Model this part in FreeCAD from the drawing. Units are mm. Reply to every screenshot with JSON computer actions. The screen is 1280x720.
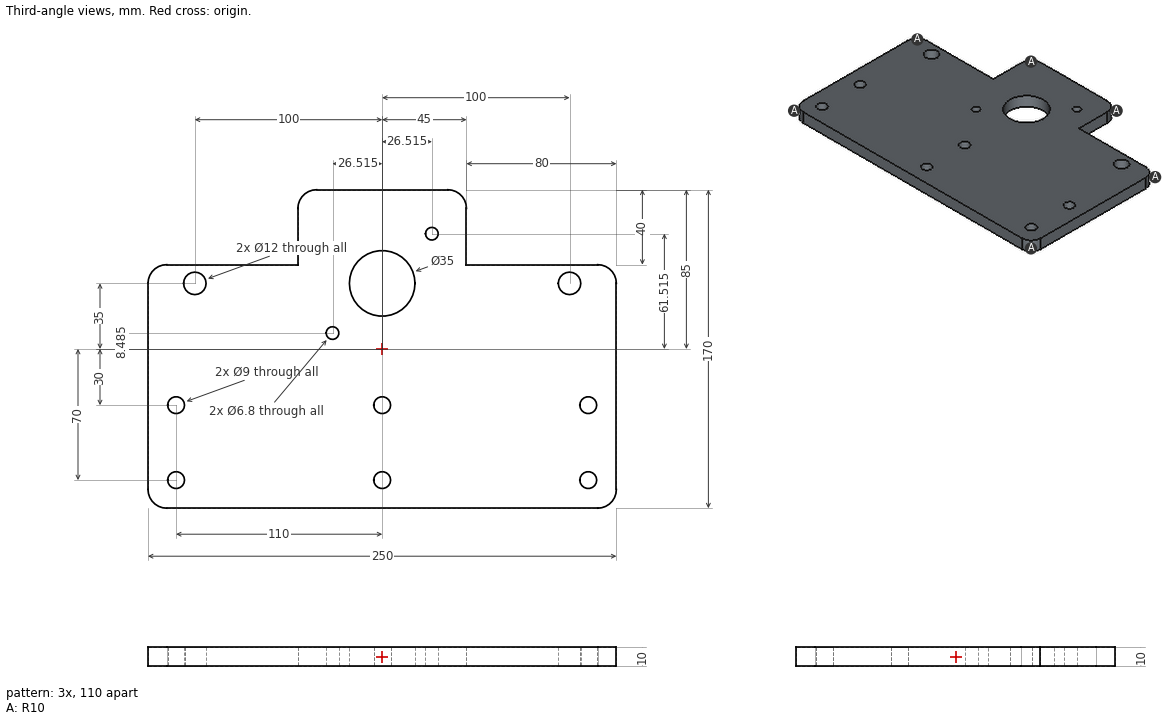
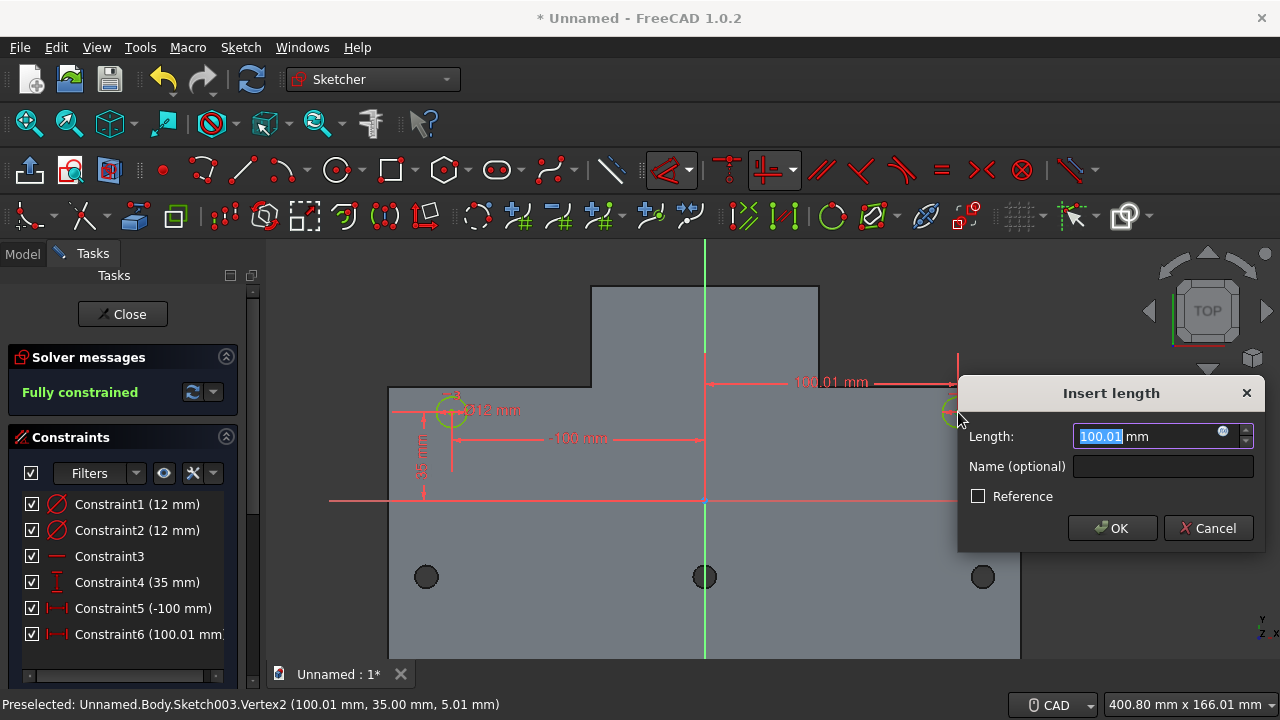
{"action": "type", "text": "100"}
{"action": "key", "text": "Return"}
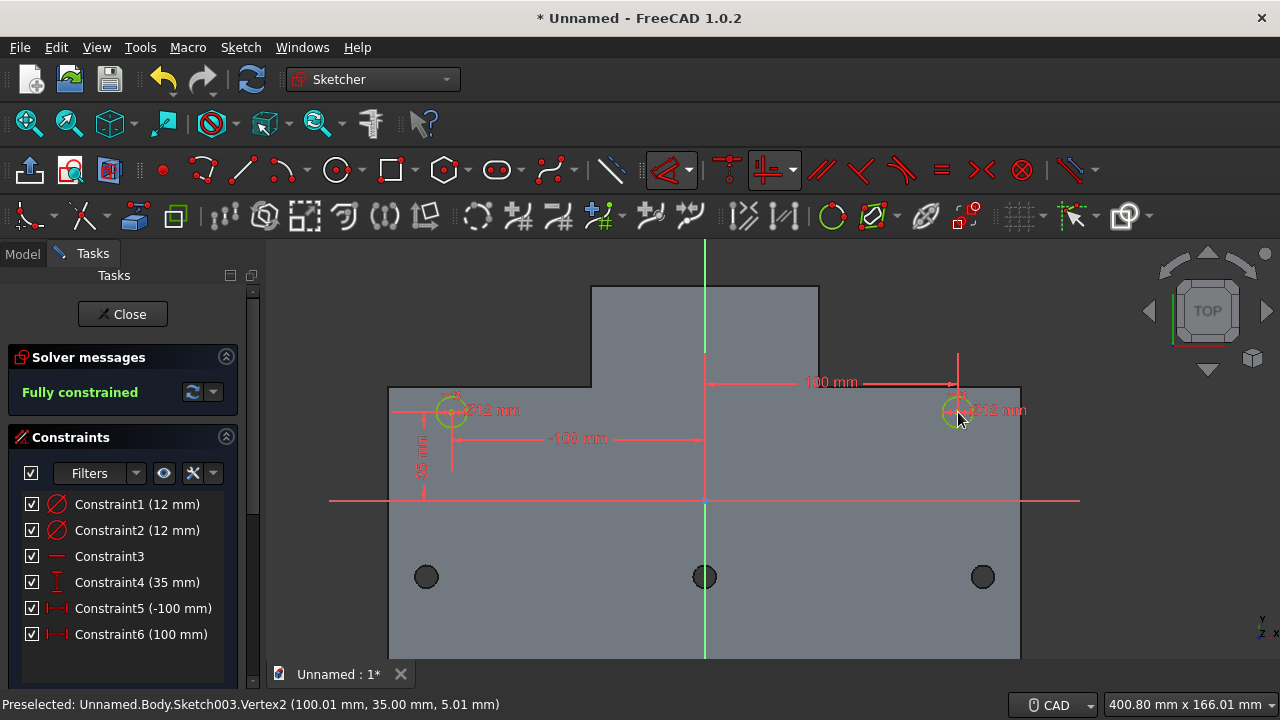
{"action": "left_click", "coordinate": [123, 314]}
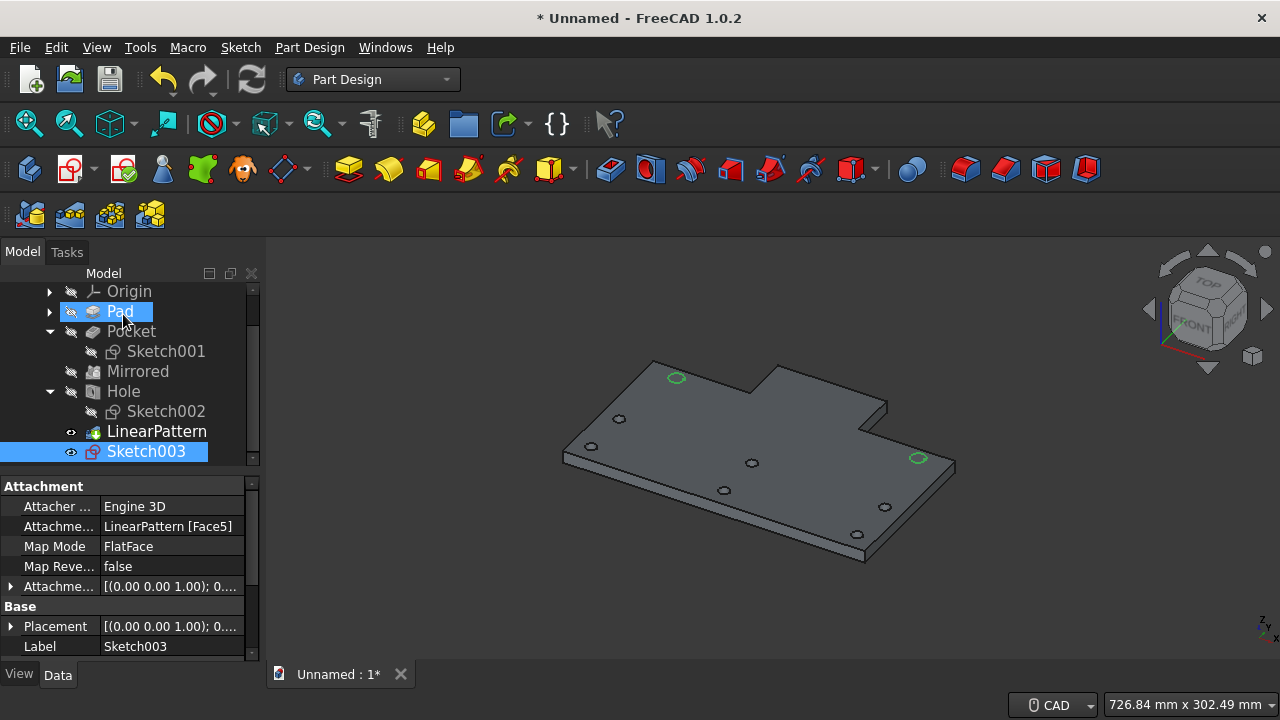
{"action": "left_click", "coordinate": [652, 170]}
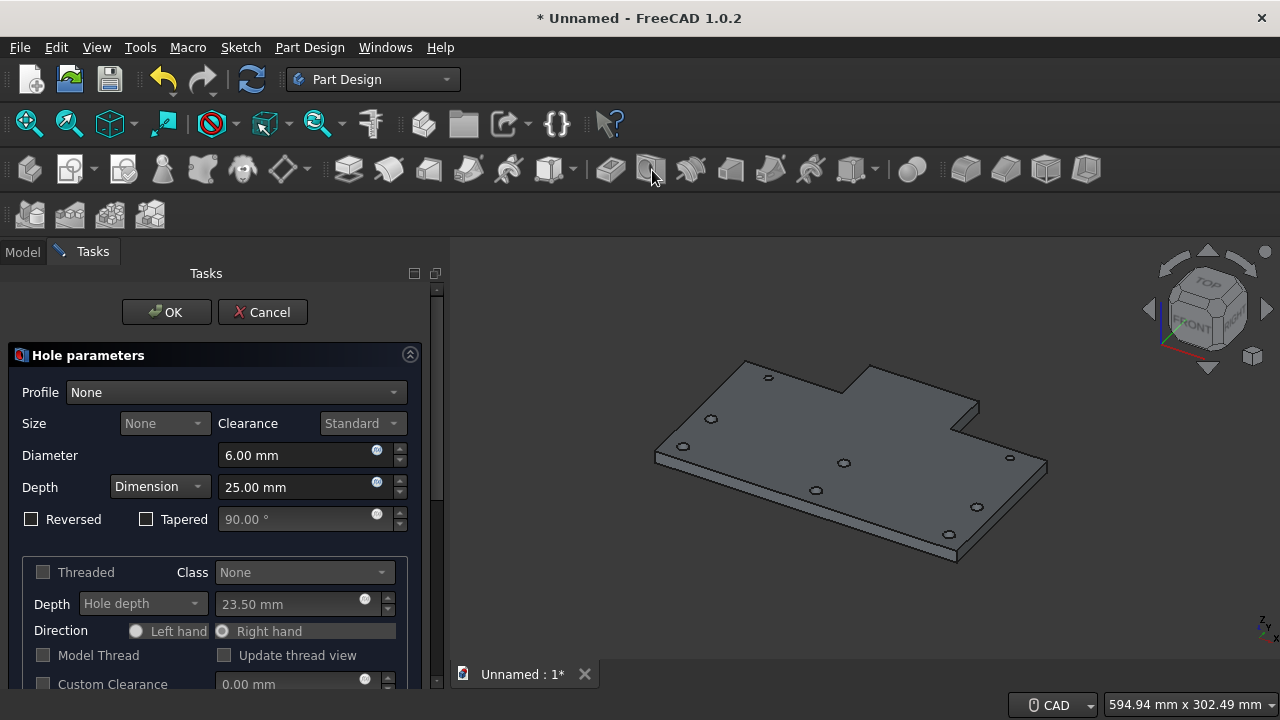
{"action": "triple_click", "coordinate": [305, 455]}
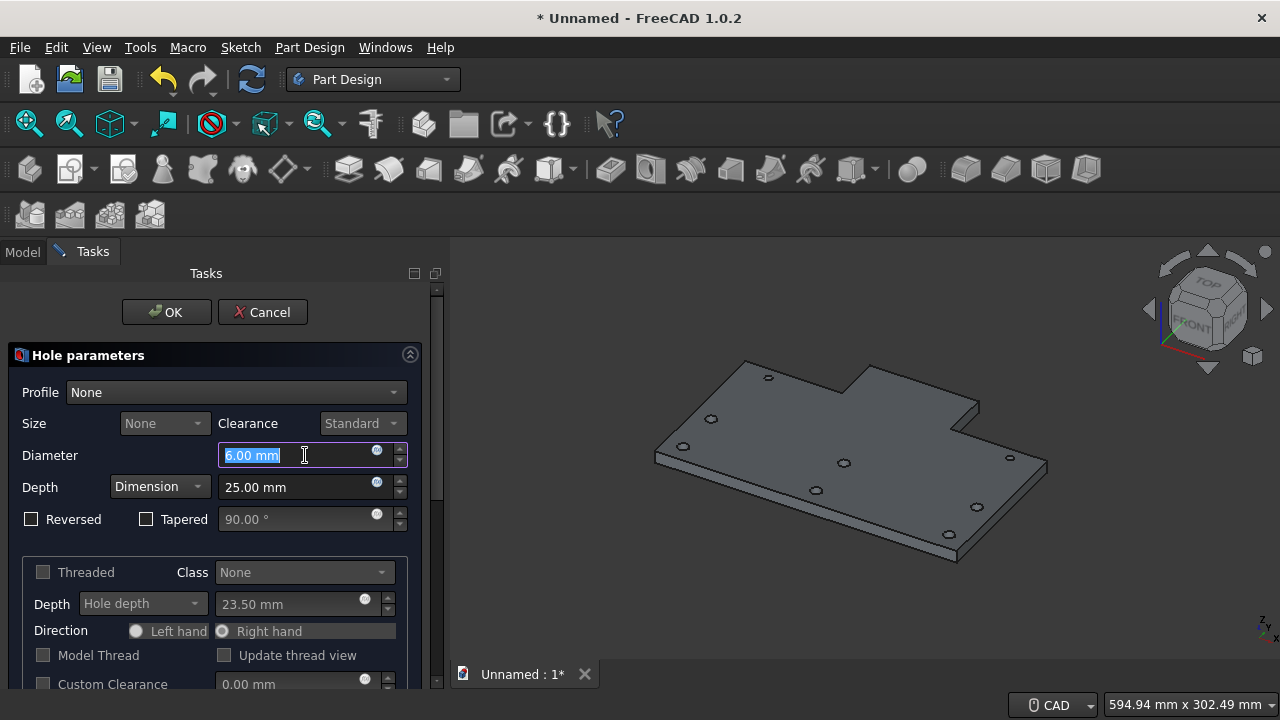
{"action": "type", "text": "12"}
{"action": "key", "text": "Tab"}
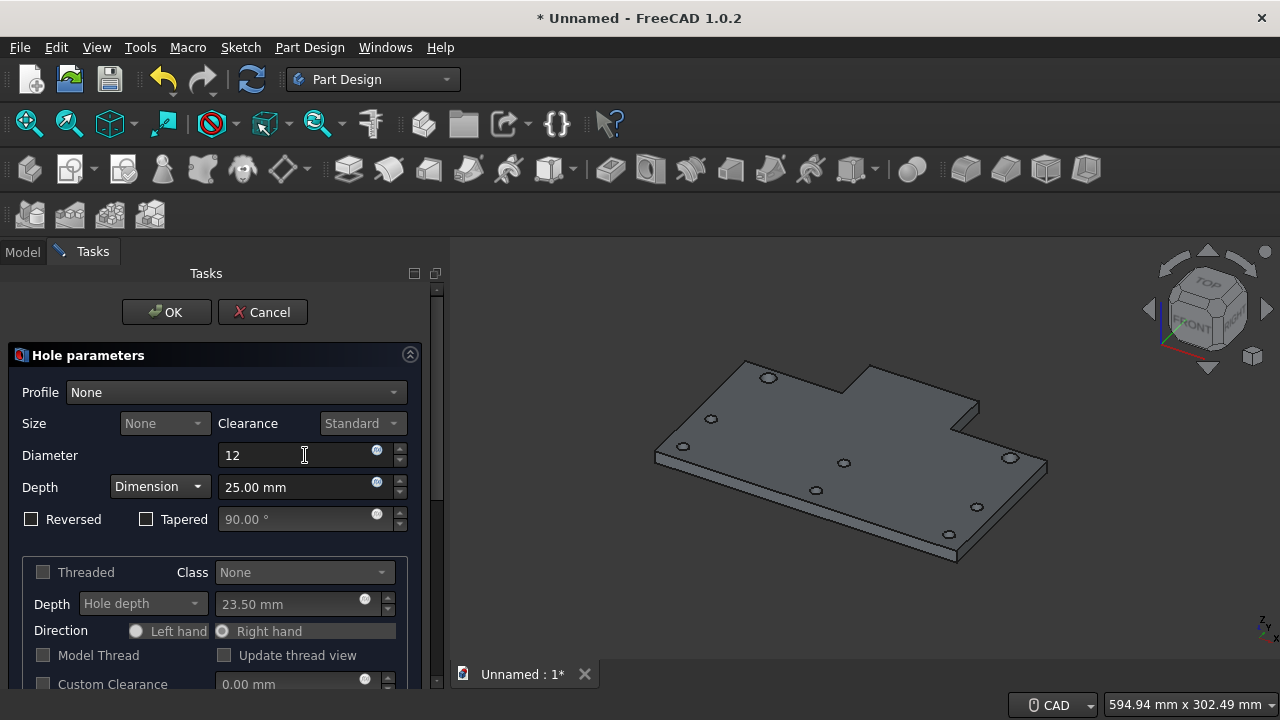
{"action": "left_click", "coordinate": [161, 486]}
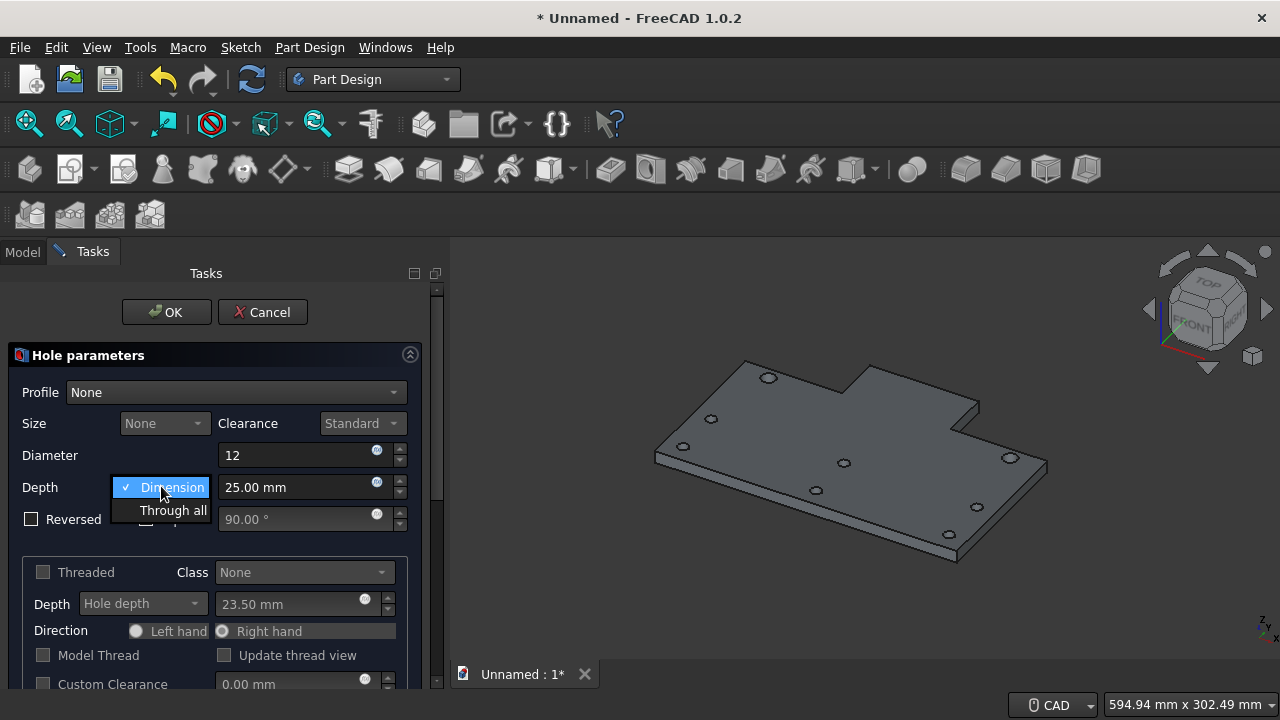
{"action": "left_click", "coordinate": [160, 510]}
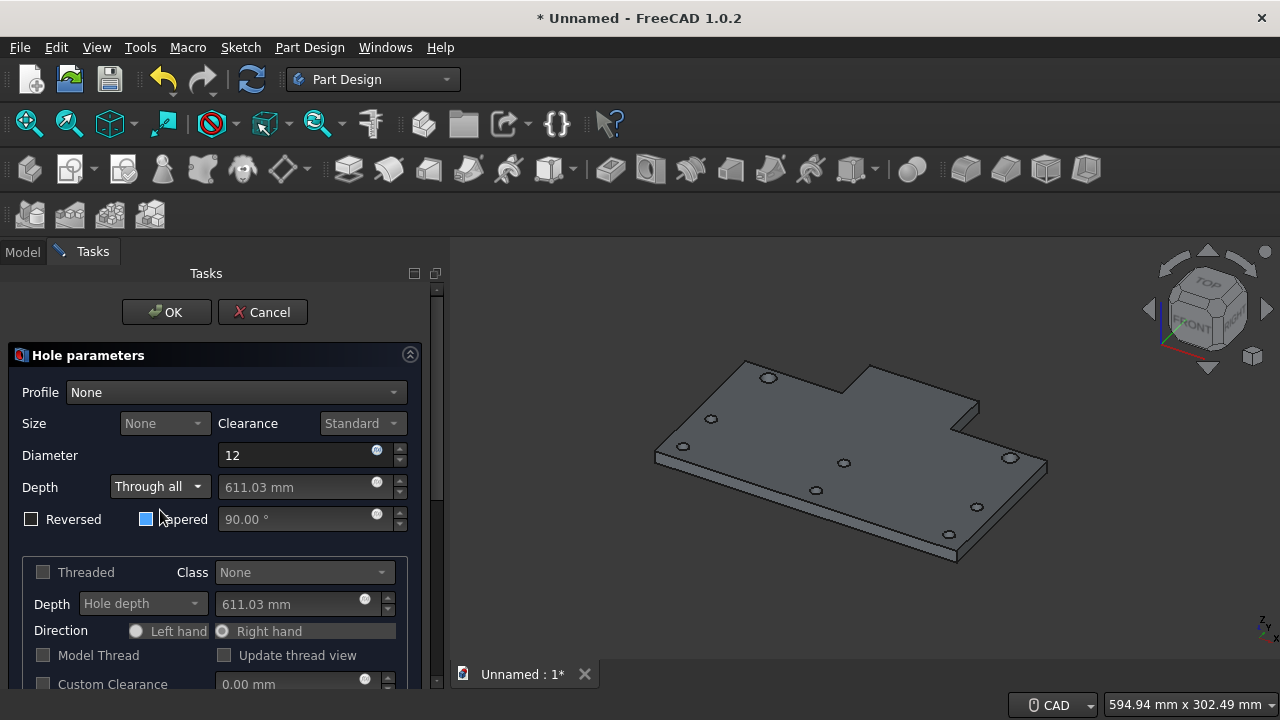
{"action": "left_click", "coordinate": [167, 312]}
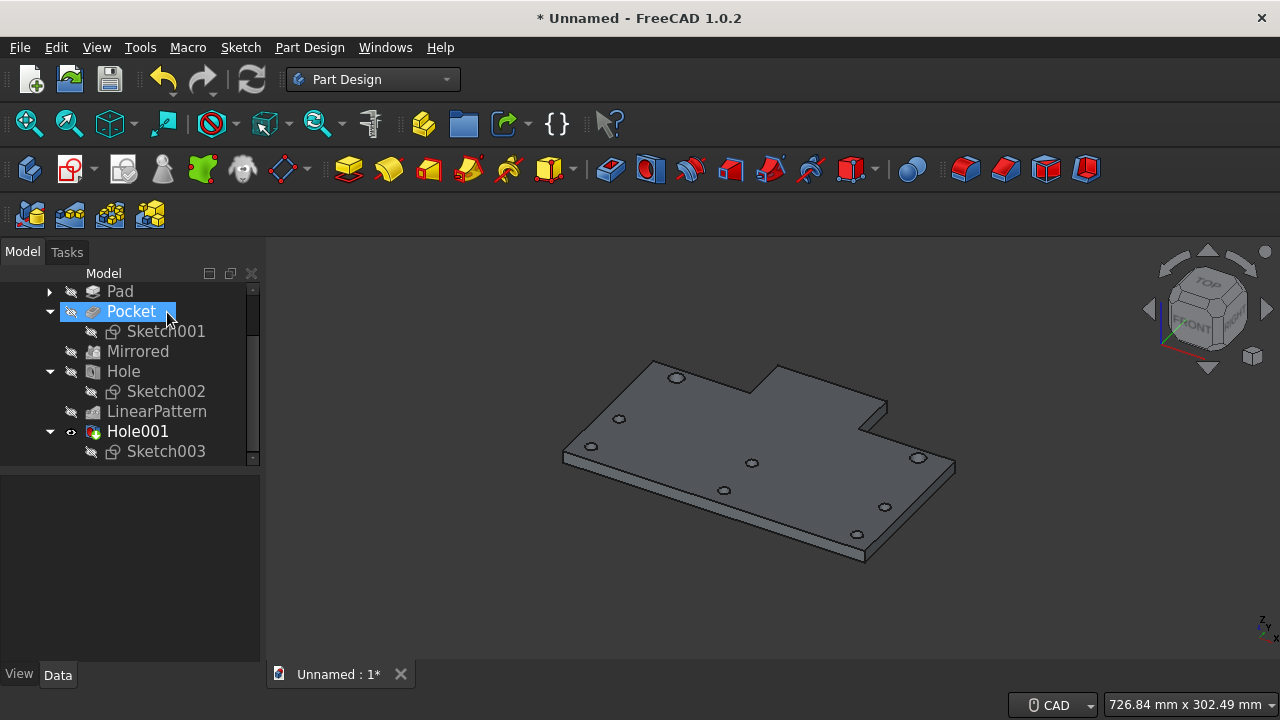
{"action": "left_click", "coordinate": [790, 424]}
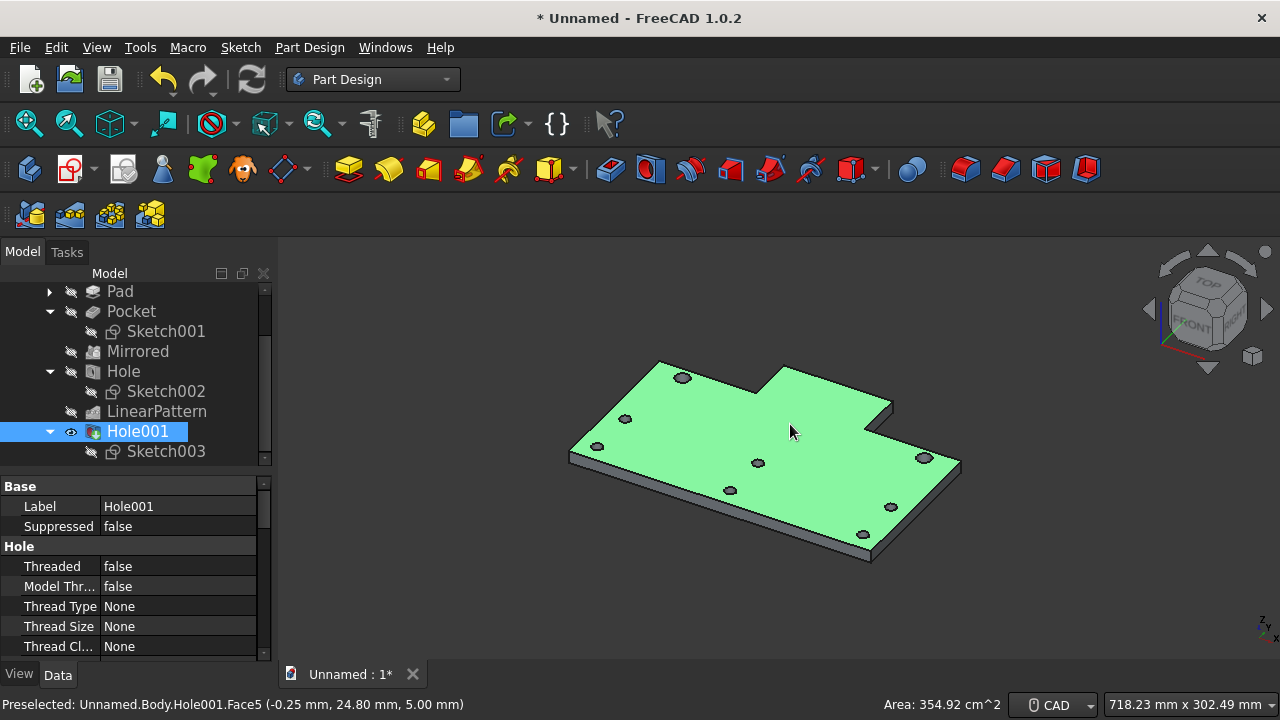
{"action": "left_click", "coordinate": [70, 170]}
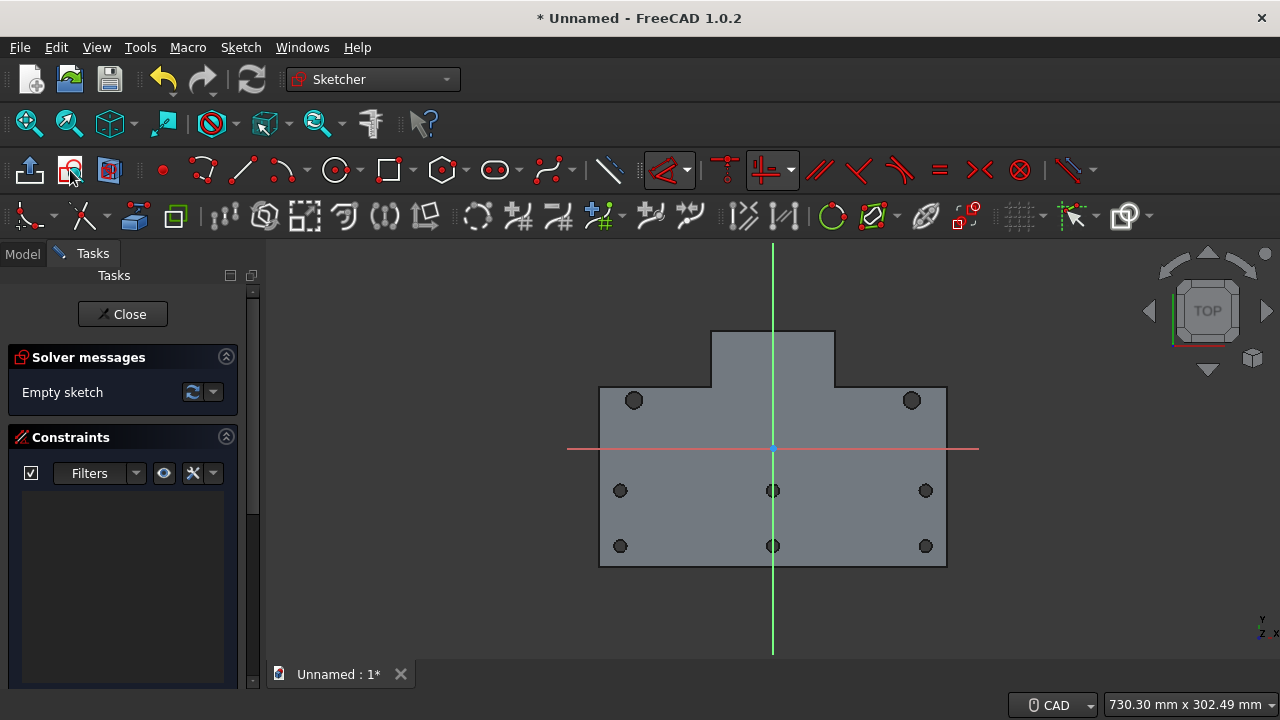
{"action": "scroll", "coordinate": [803, 397], "scroll_direction": "up", "scroll_amount": 6}